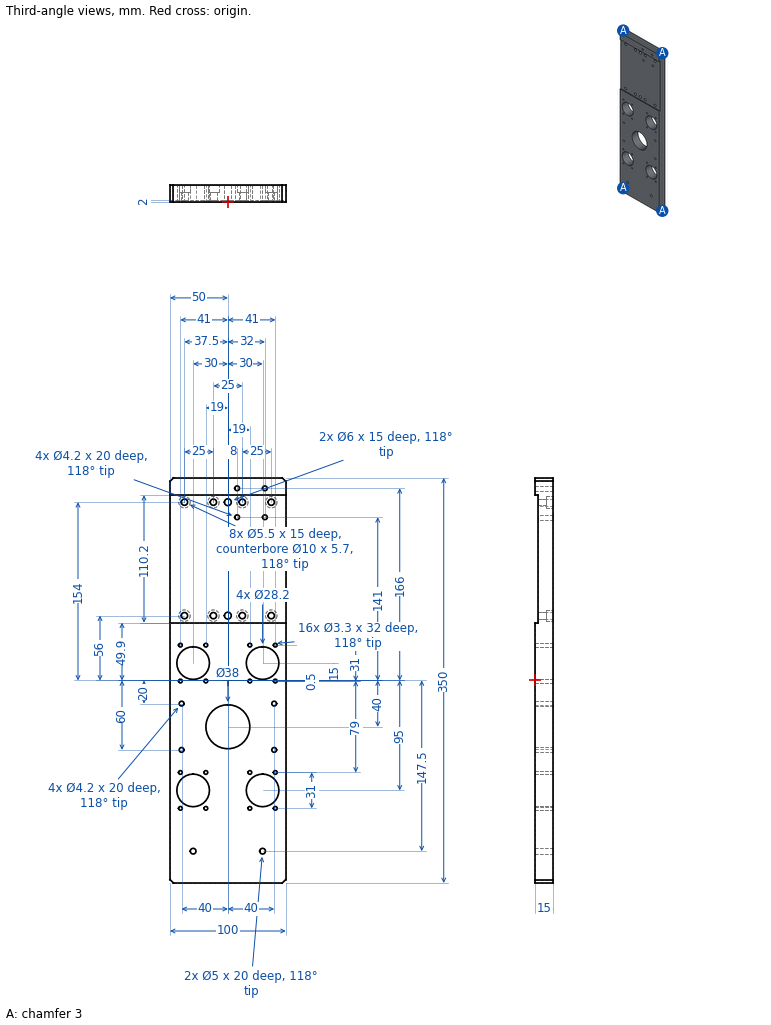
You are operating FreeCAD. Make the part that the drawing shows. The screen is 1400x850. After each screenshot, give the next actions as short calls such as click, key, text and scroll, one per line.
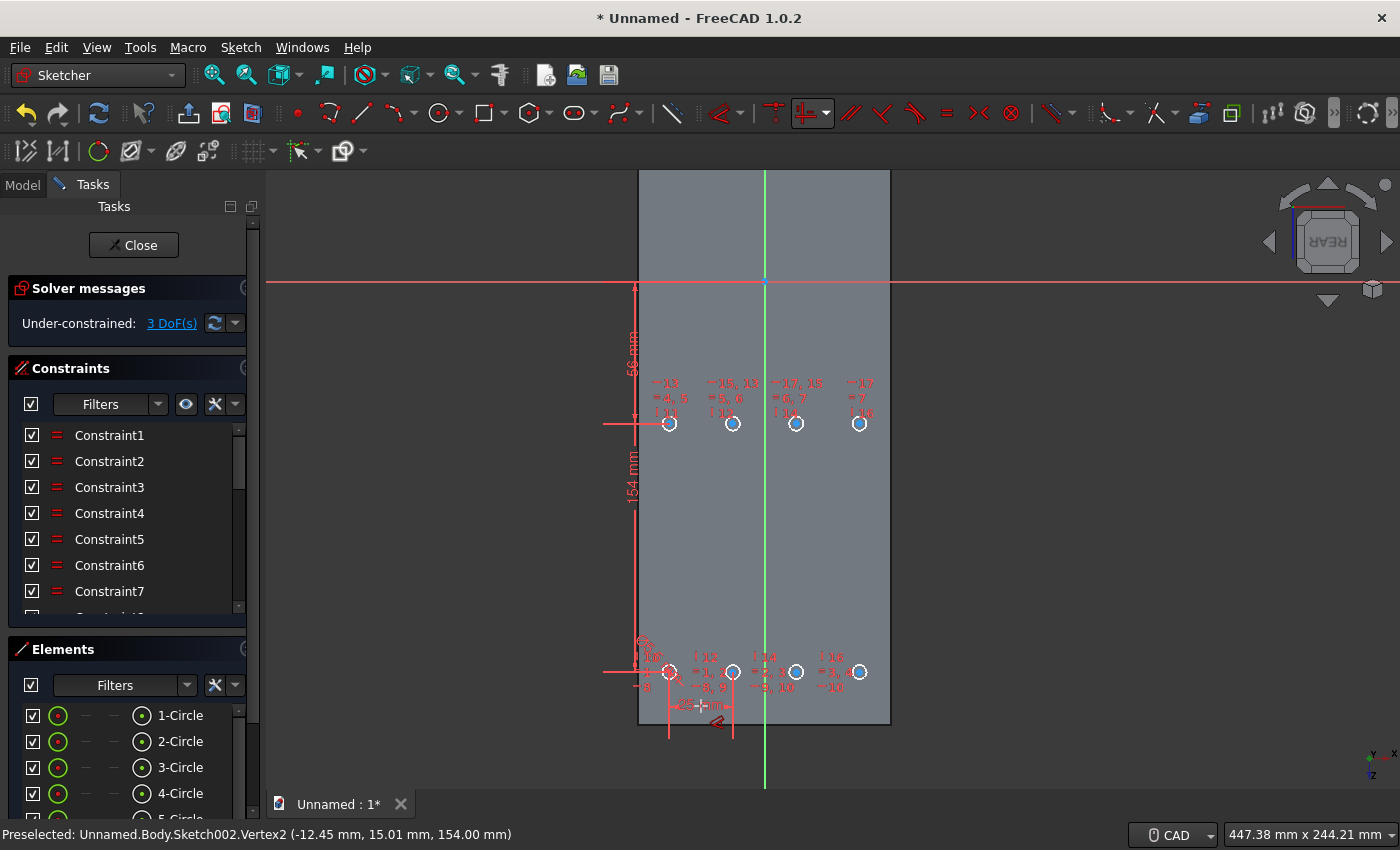
click(733, 672)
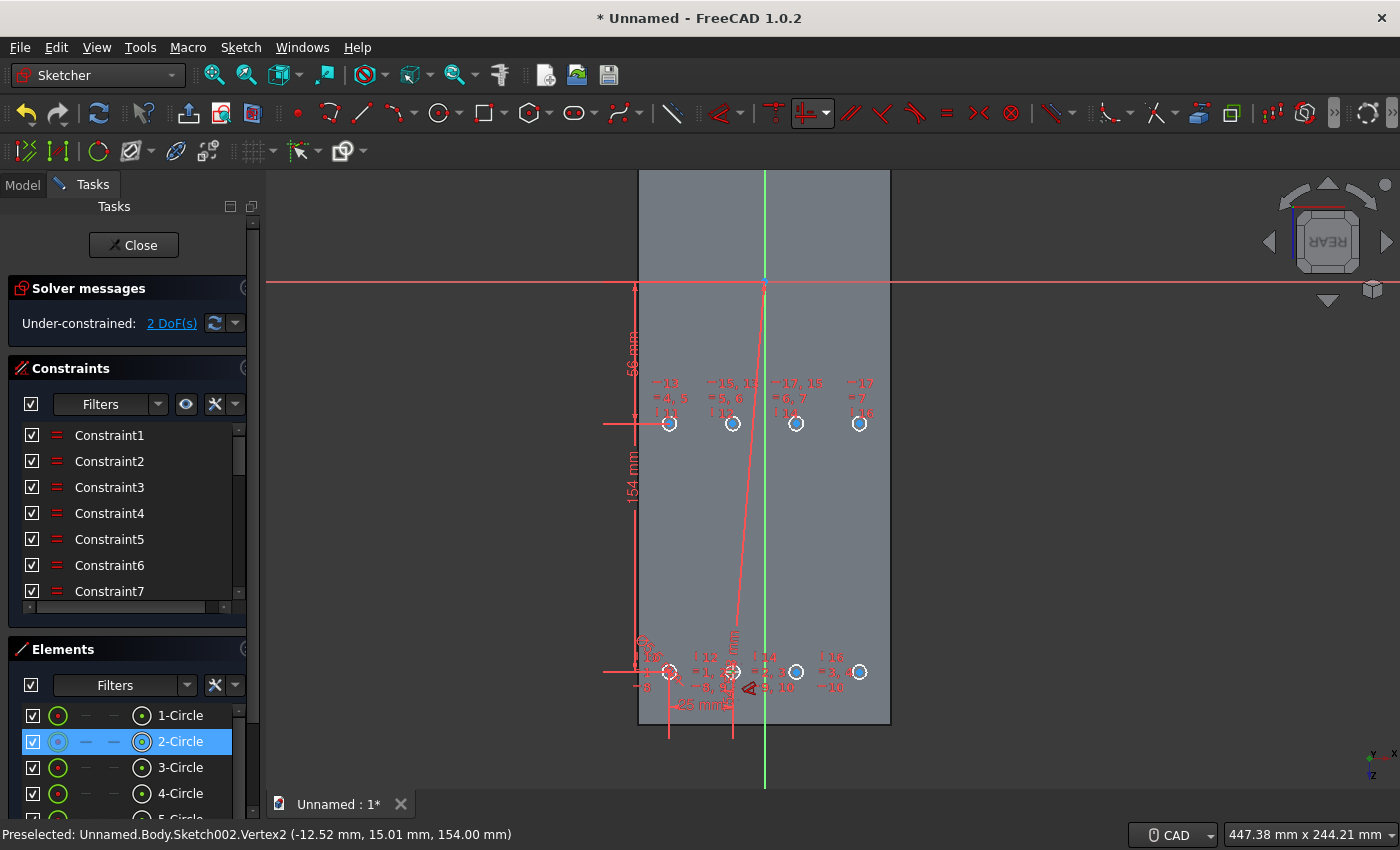
click(796, 672)
click(779, 706)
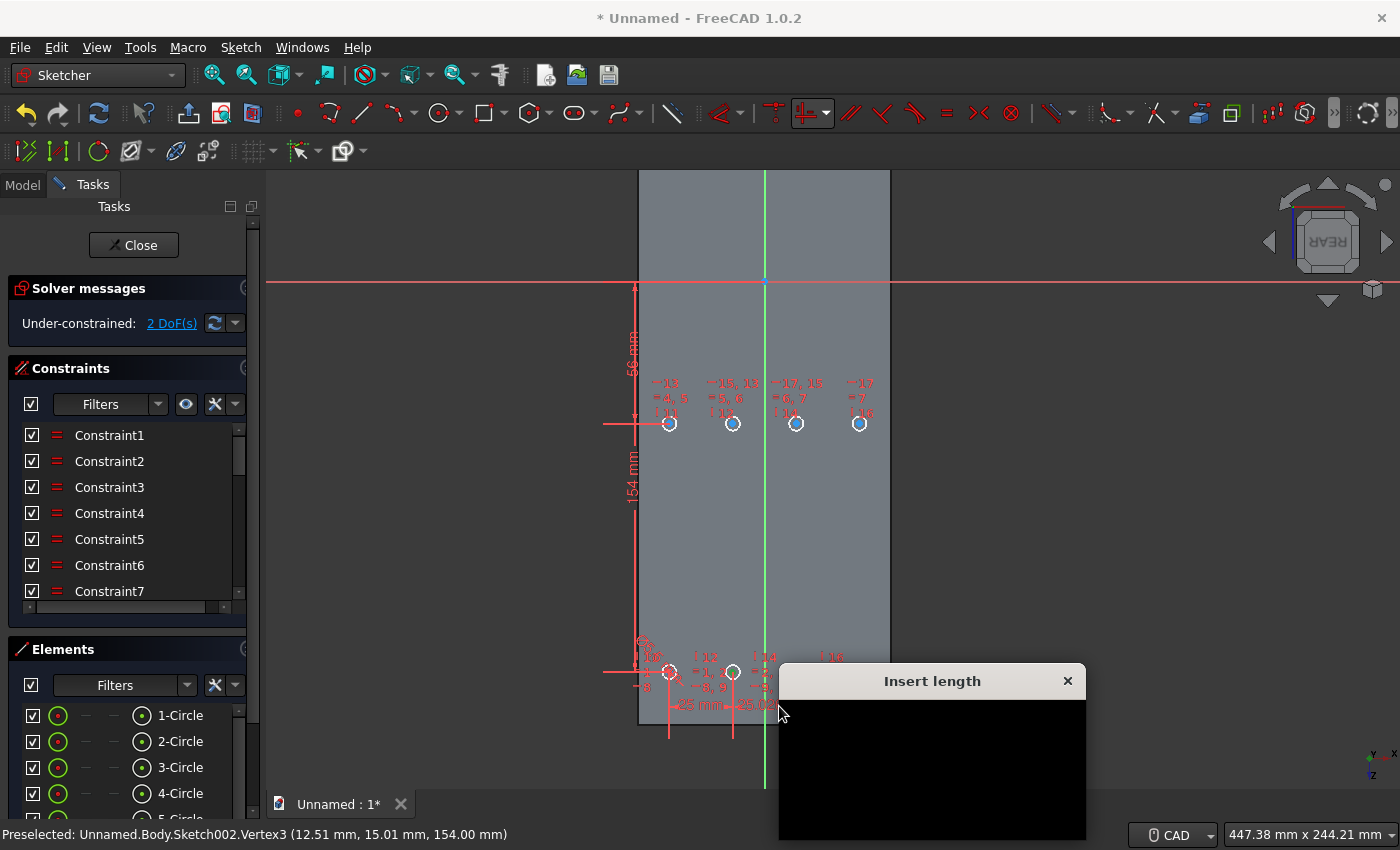
text(25)
key(Return)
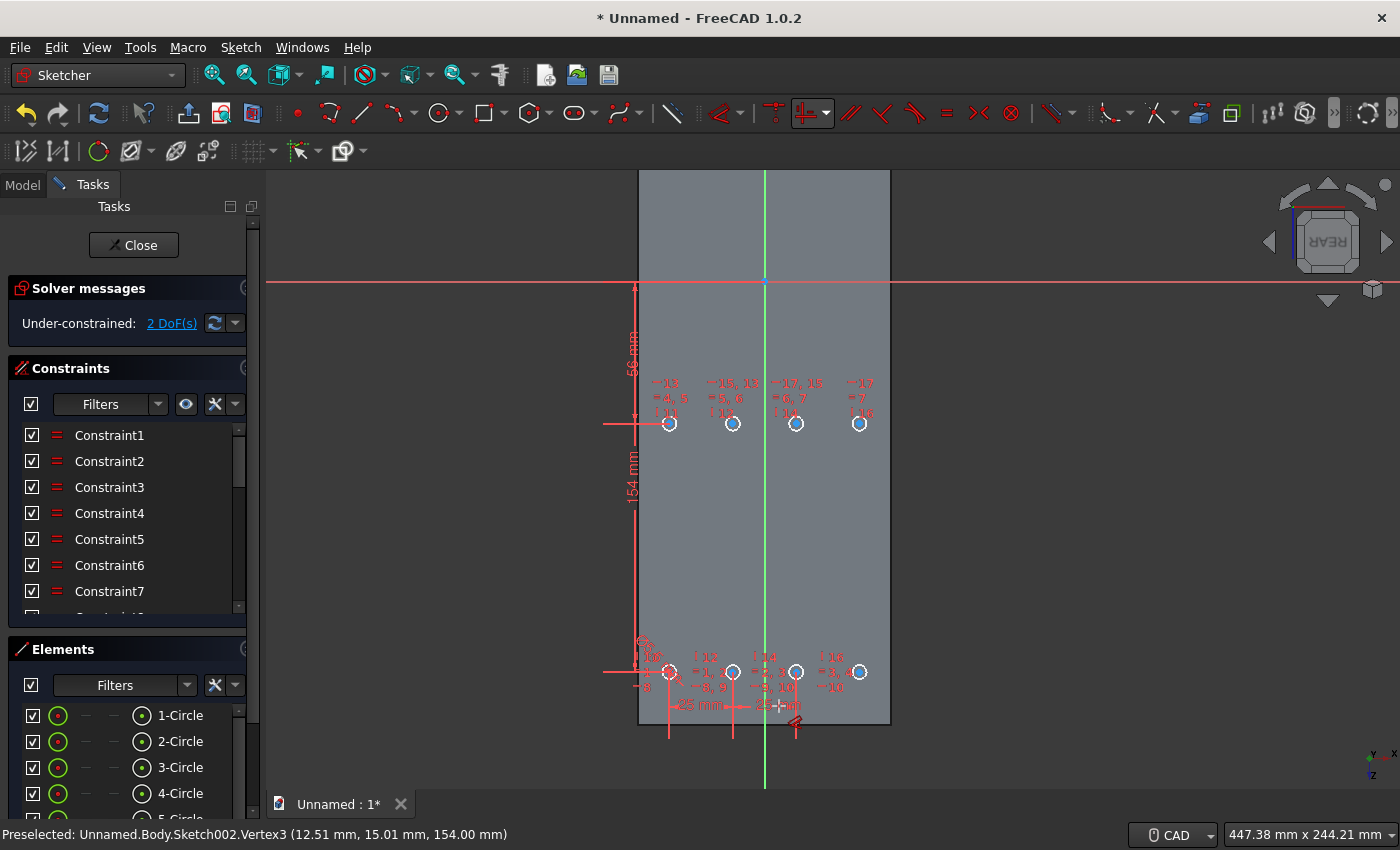
click(796, 672)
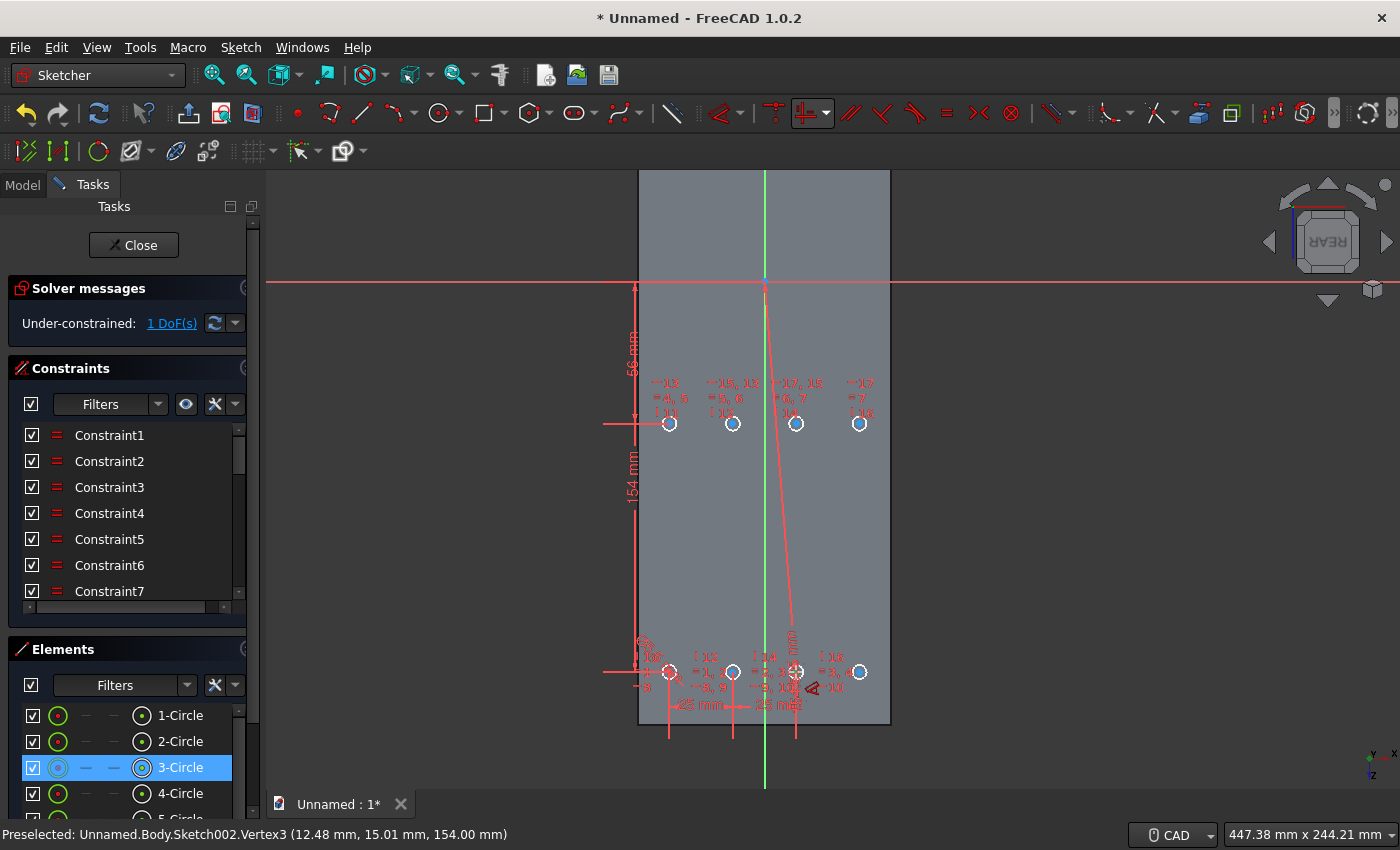
click(860, 672)
click(850, 706)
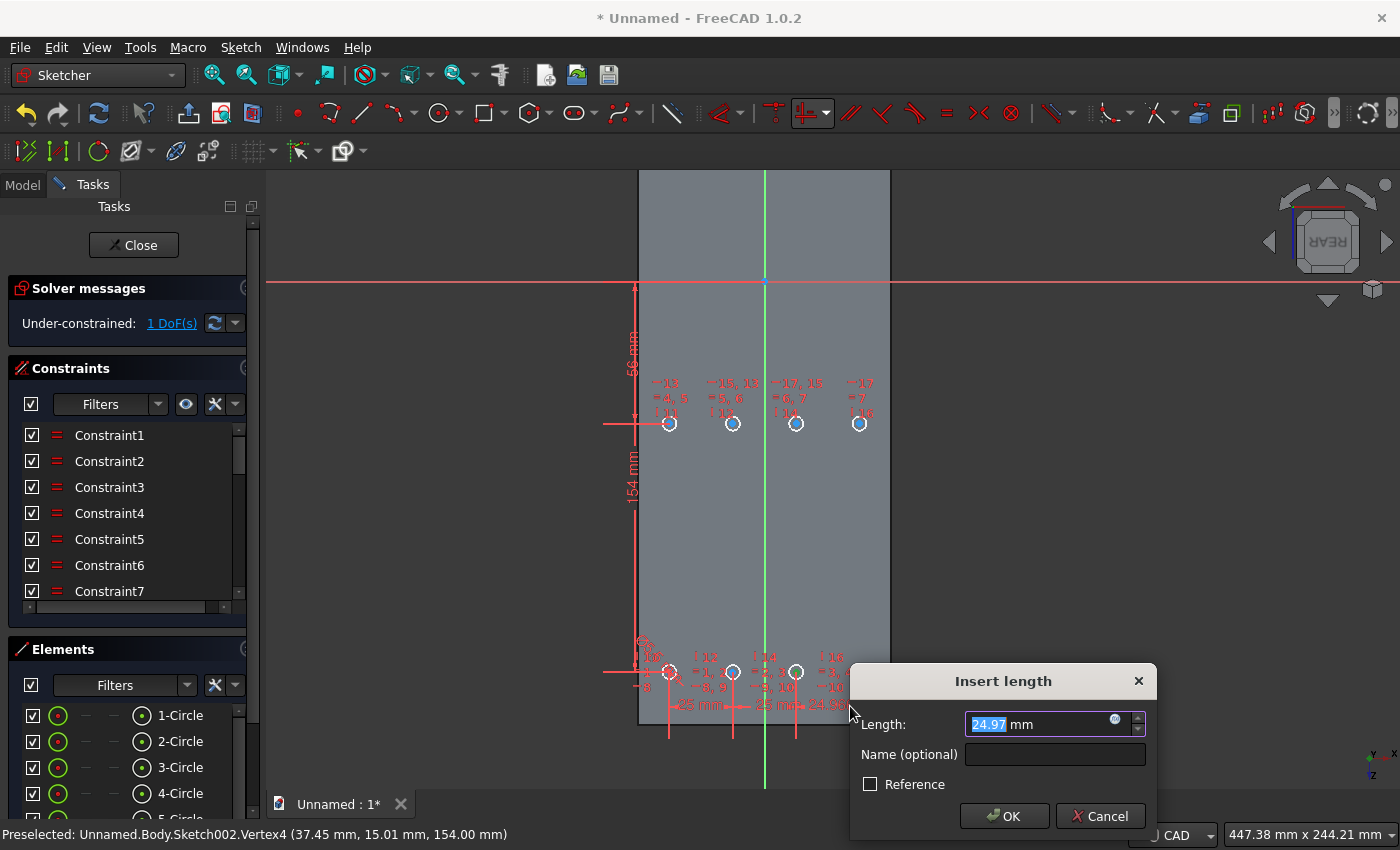
text(25)
key(Return)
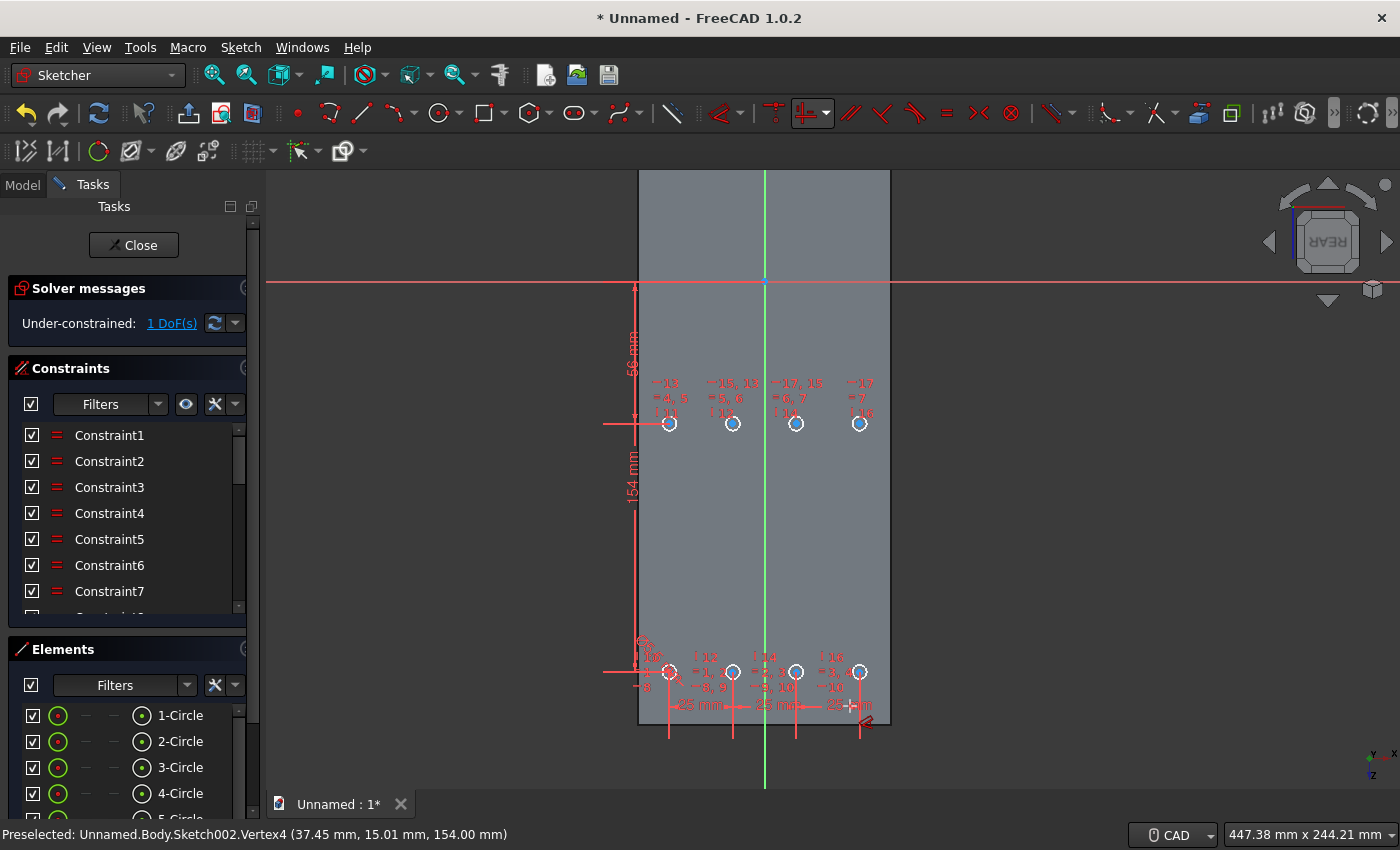
click(669, 672)
click(717, 248)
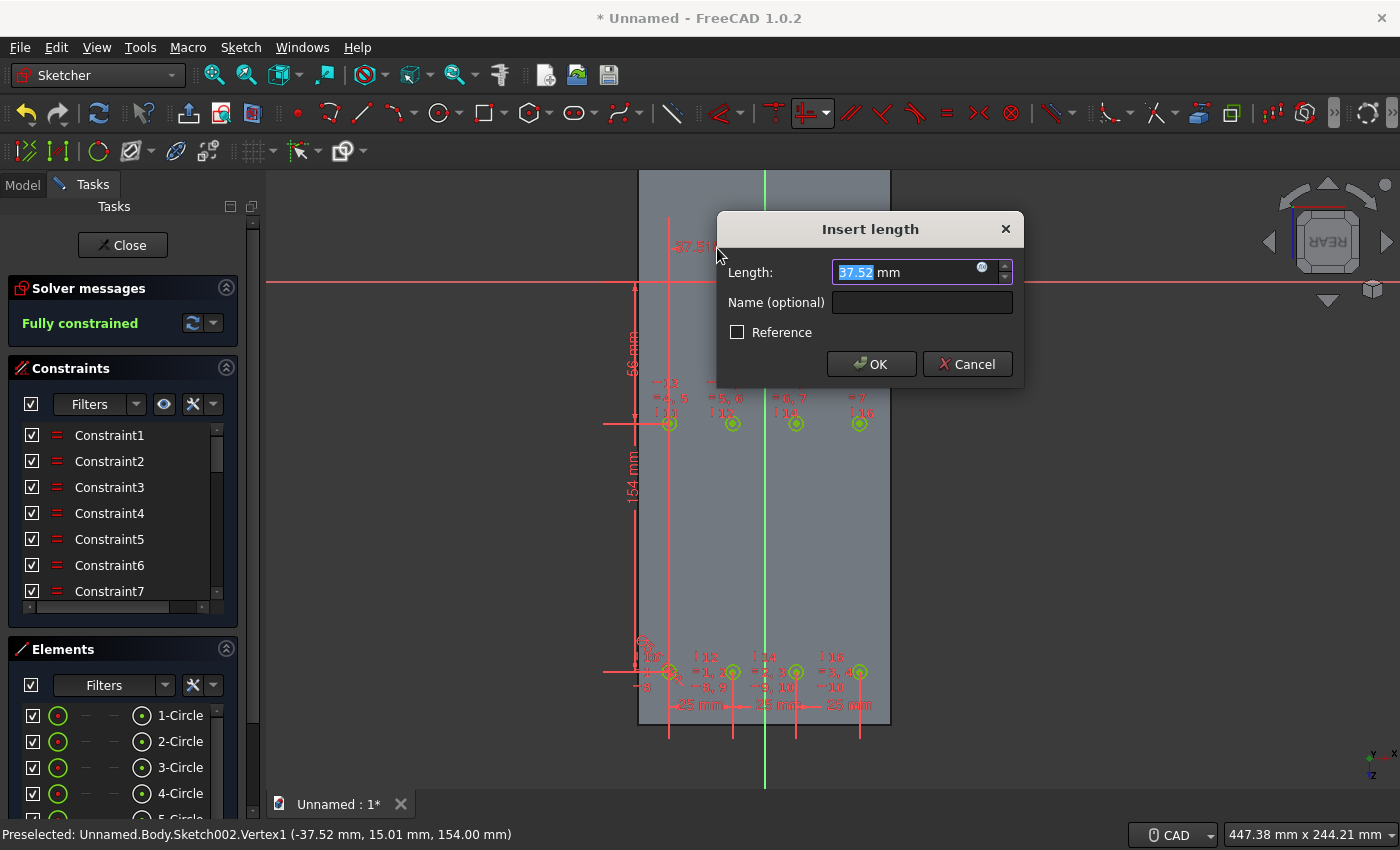
text(37.5)
key(Return)
key(Escape)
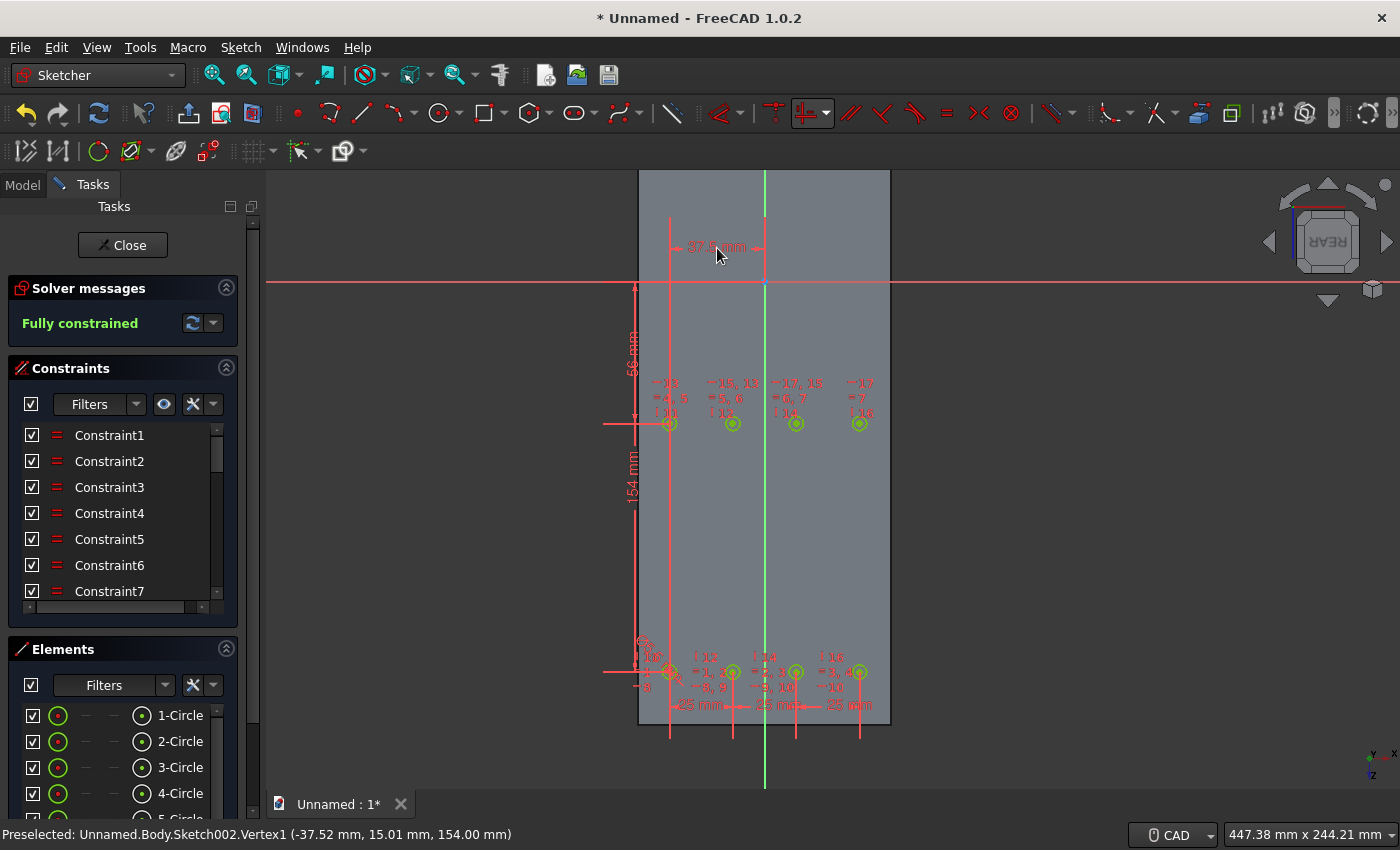
click(123, 245)